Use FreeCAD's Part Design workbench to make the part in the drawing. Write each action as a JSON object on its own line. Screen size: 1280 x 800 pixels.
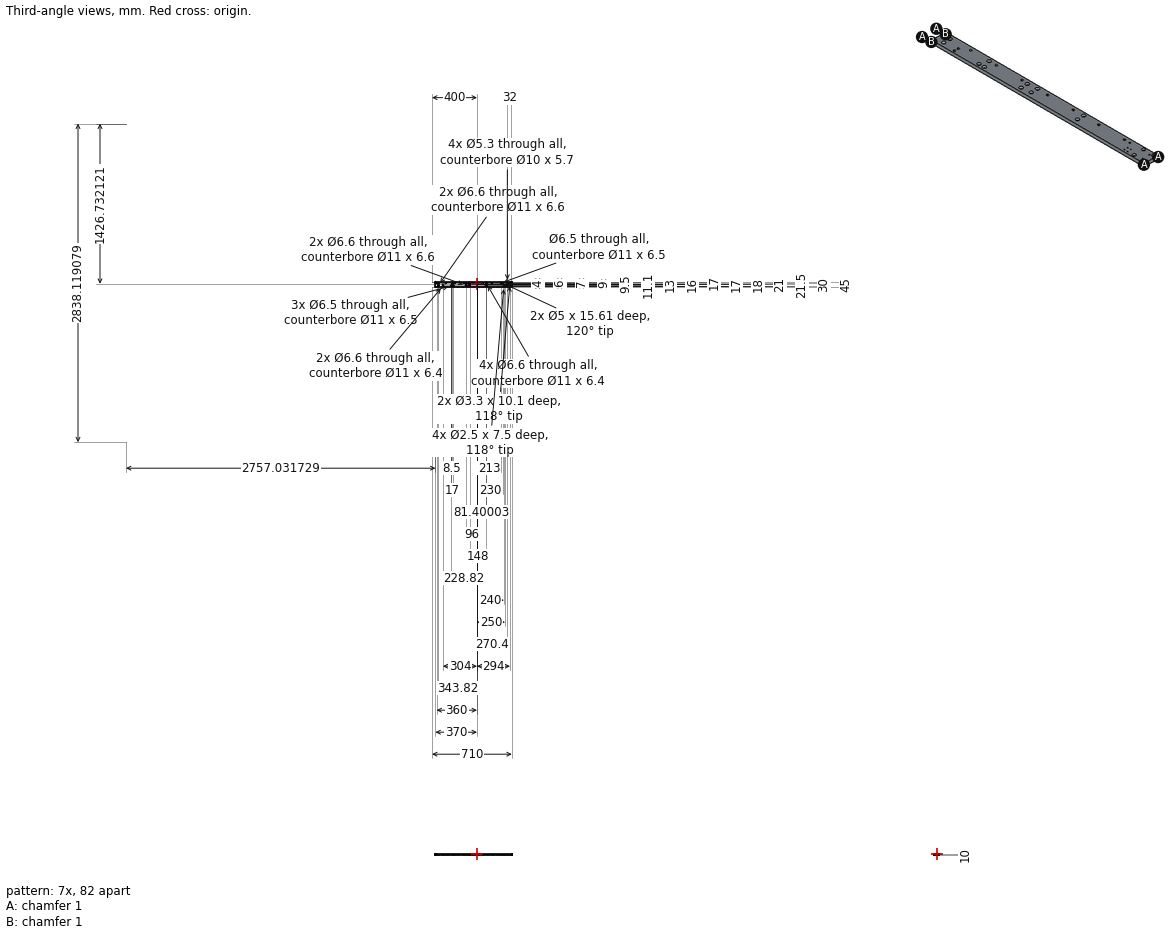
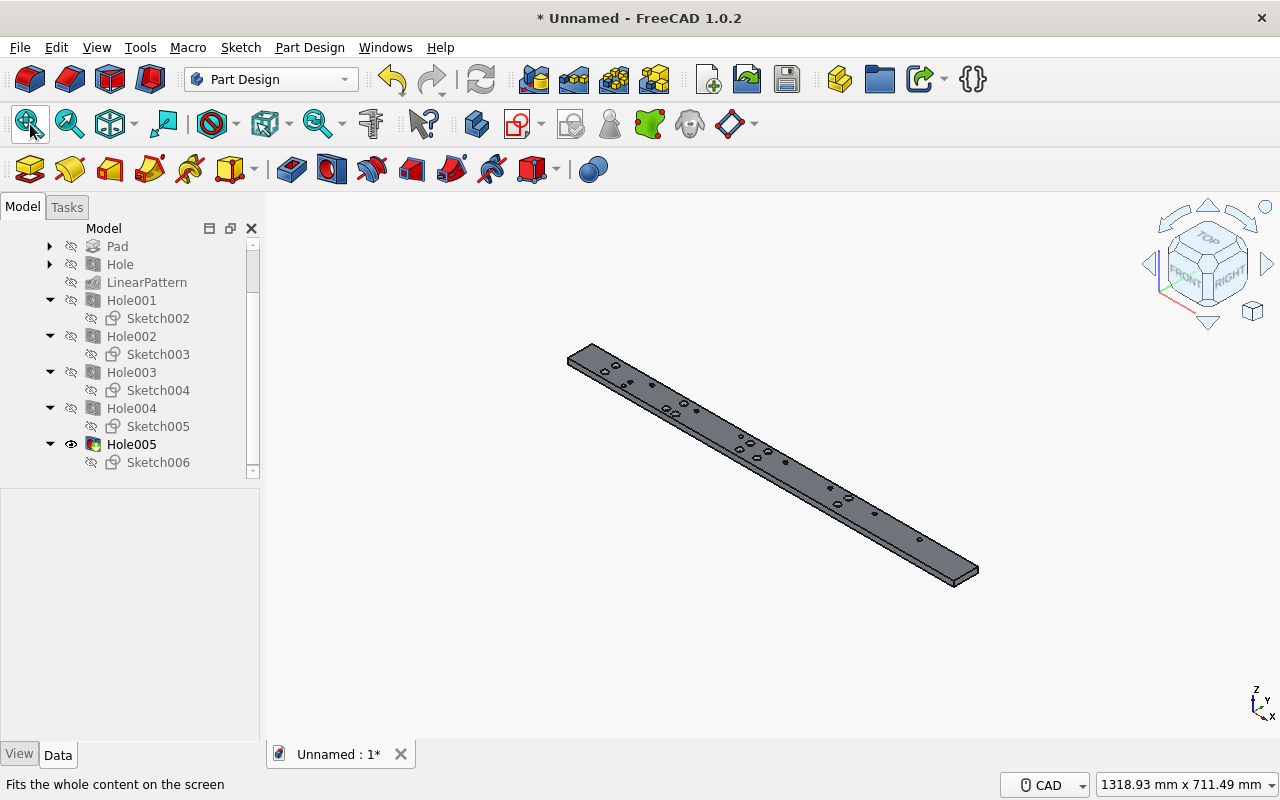
{"action": "left_click", "coordinate": [30, 124]}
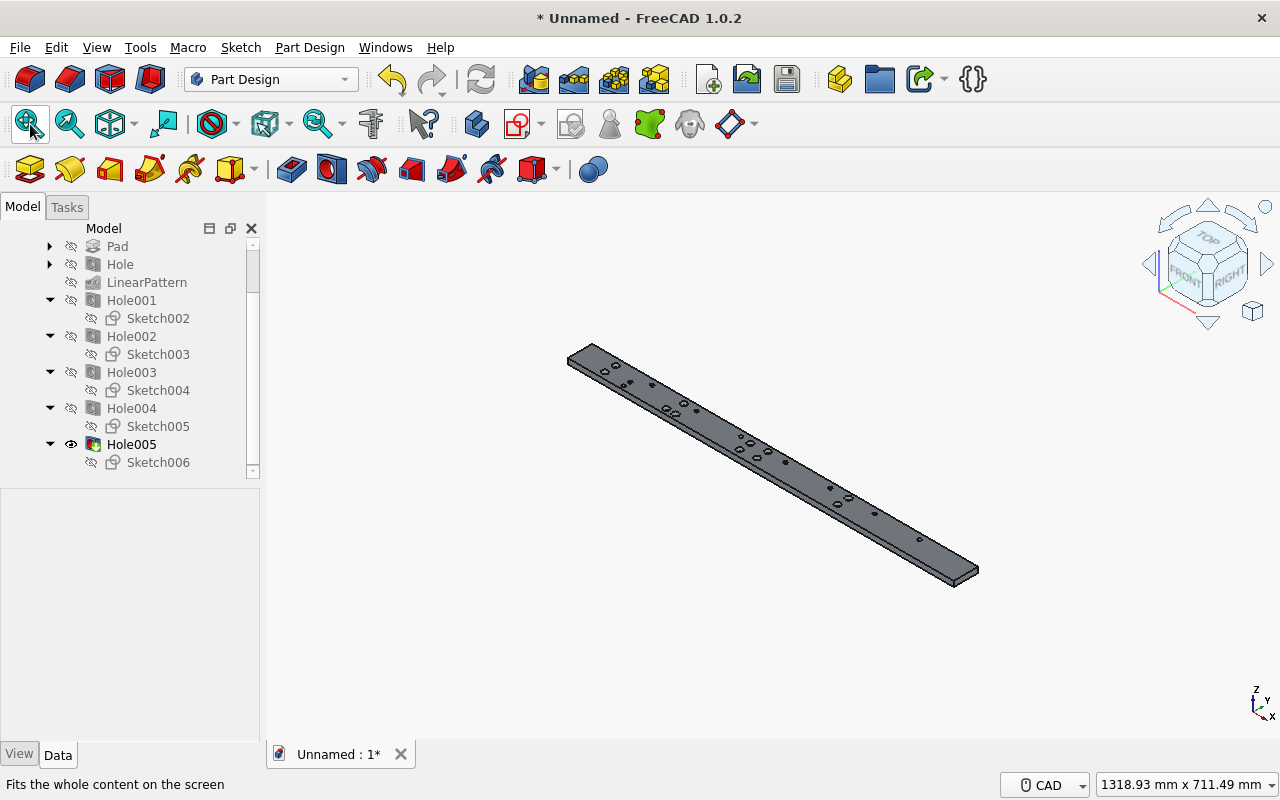
{"action": "scroll", "coordinate": [592, 346], "scroll_direction": "up", "scroll_amount": 9}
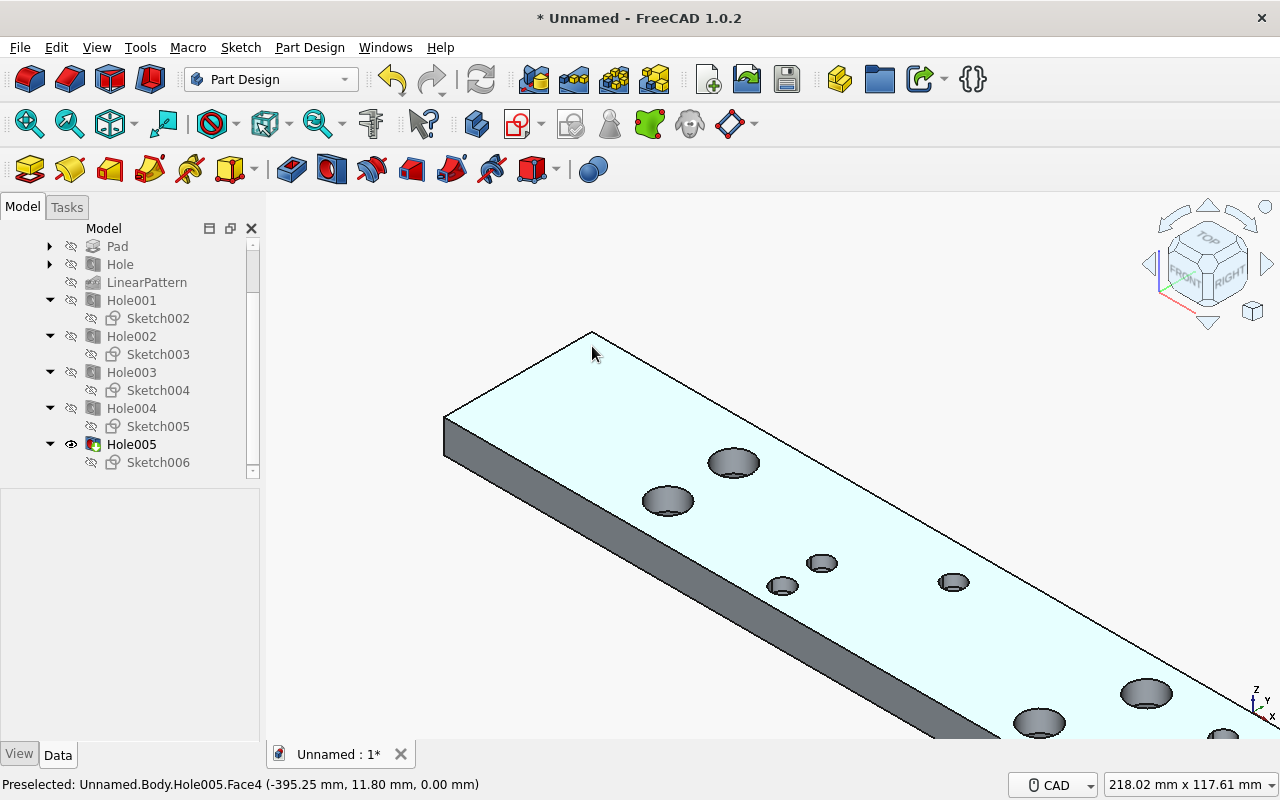
{"action": "left_click", "coordinate": [30, 124]}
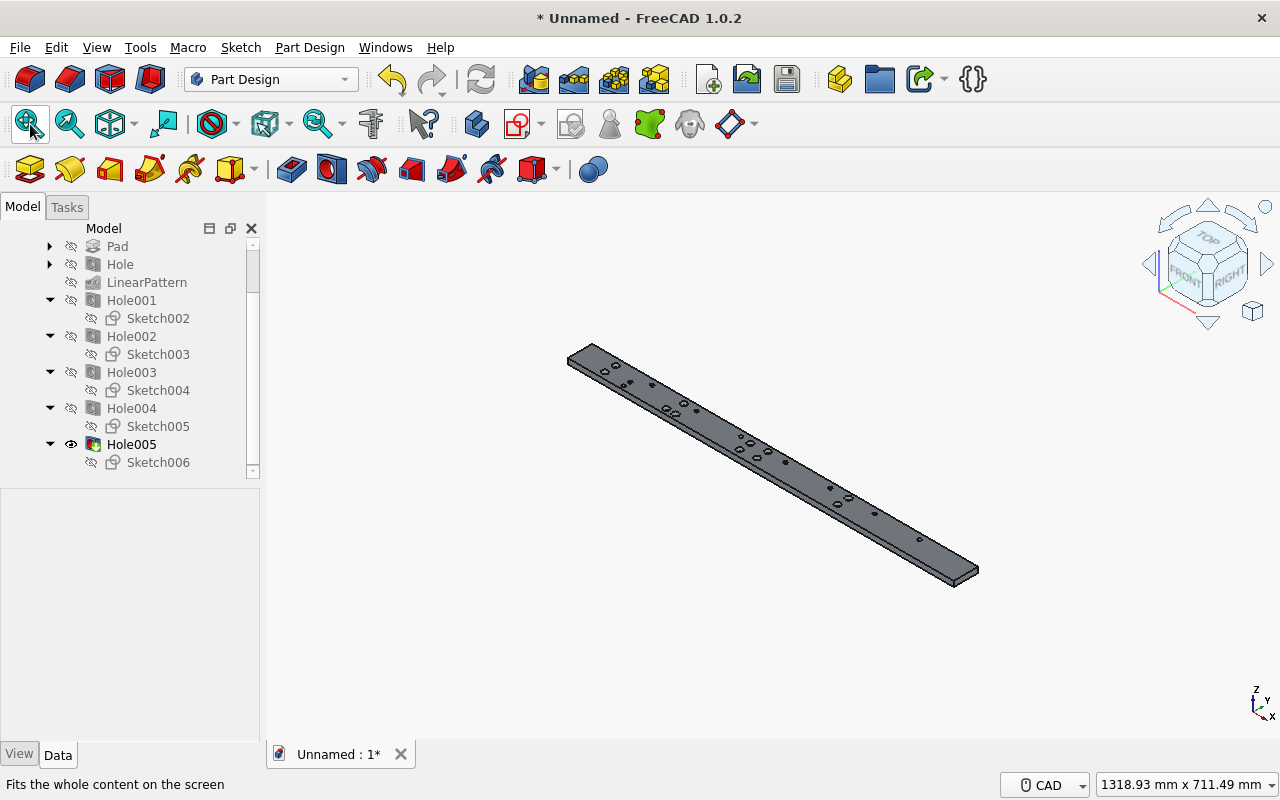
{"action": "key", "text": "1"}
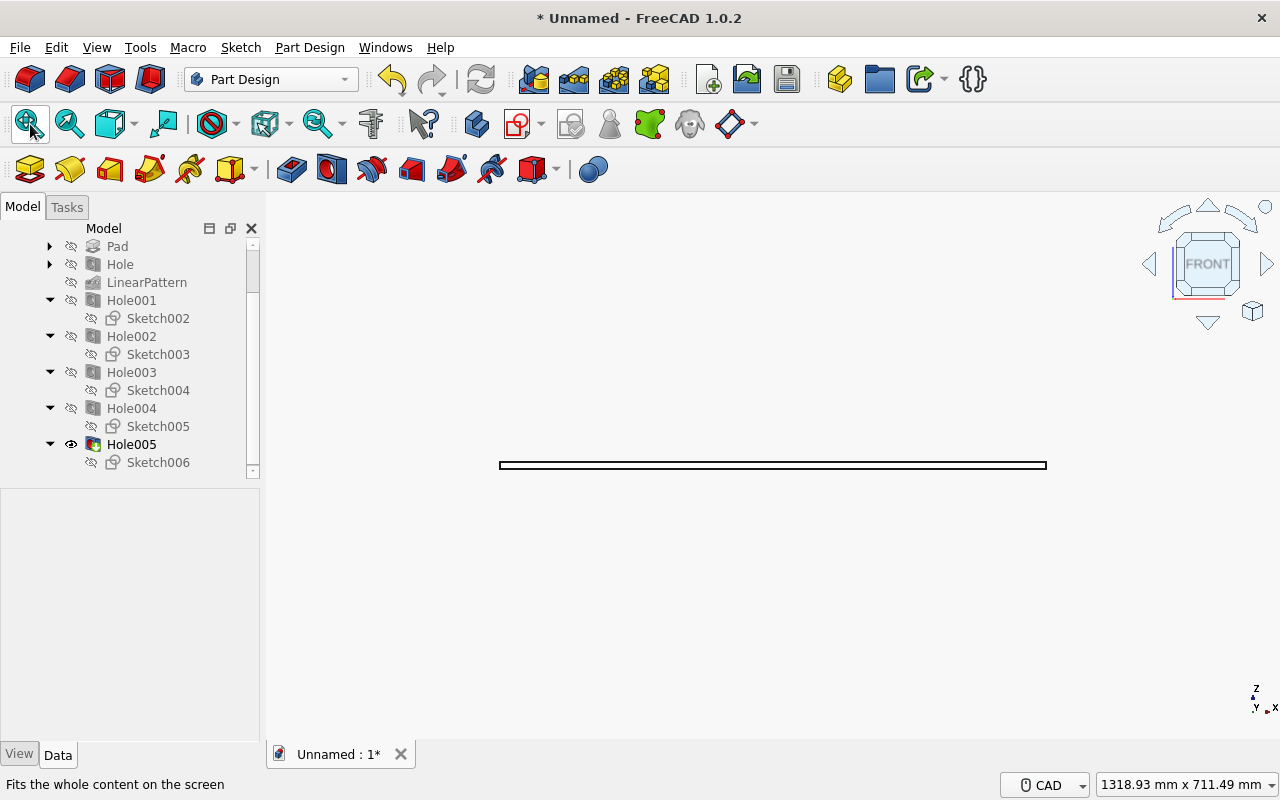
{"action": "scroll", "coordinate": [500, 465], "scroll_direction": "up", "scroll_amount": 9}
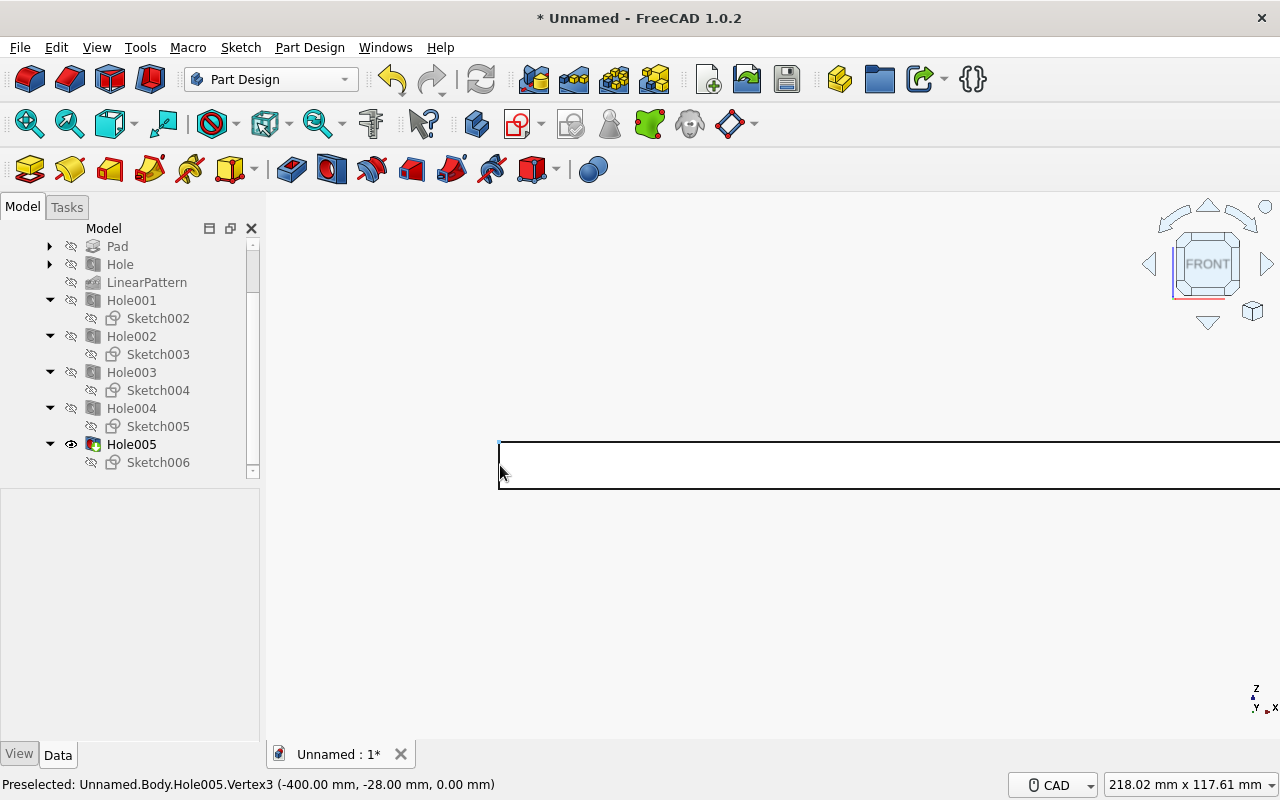
{"action": "left_click", "coordinate": [499, 465]}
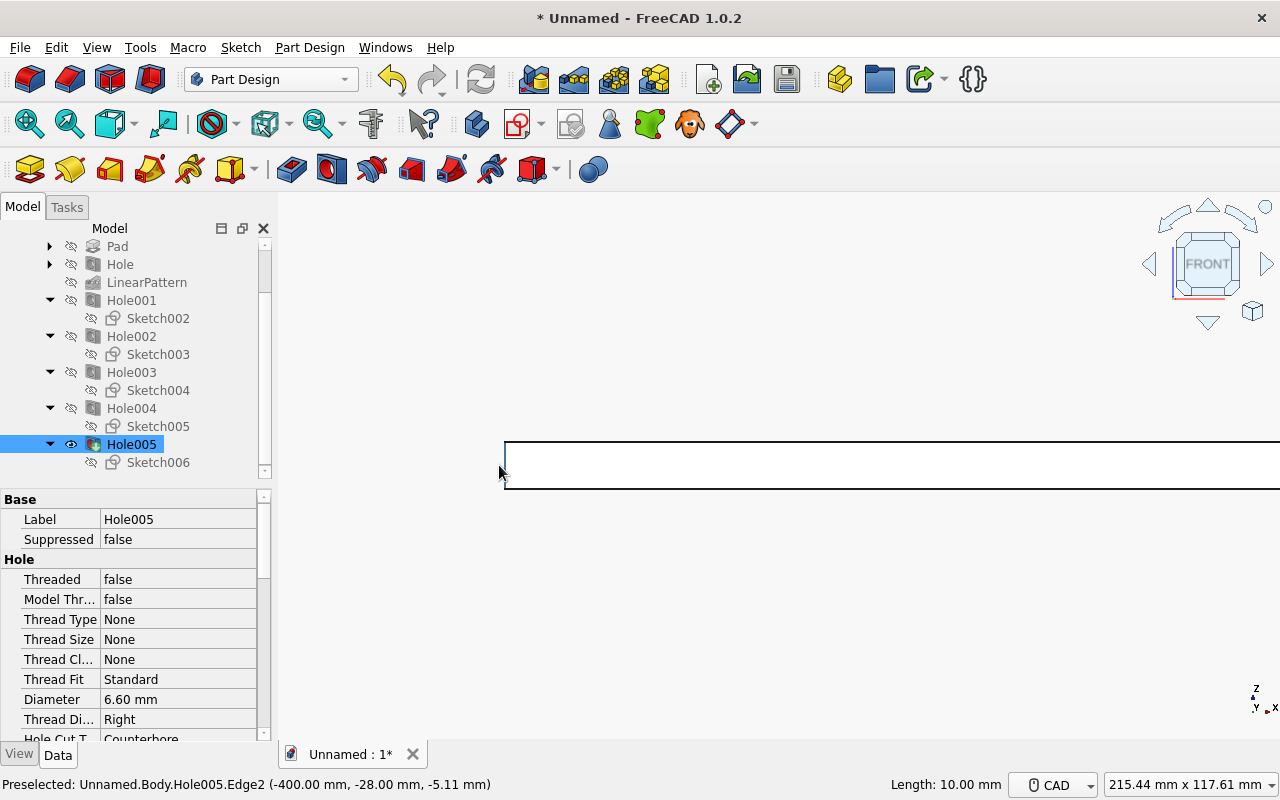
{"action": "left_click", "coordinate": [30, 124]}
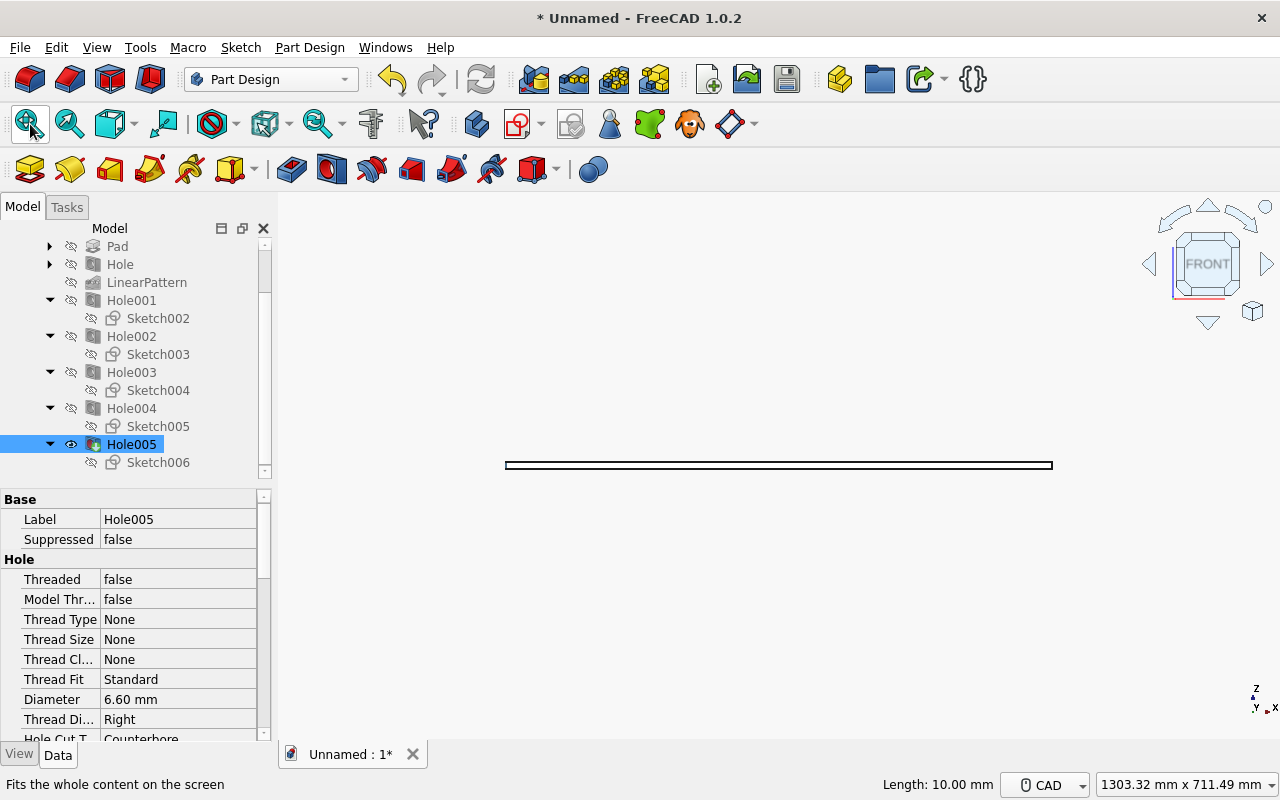
{"action": "key", "text": "3"}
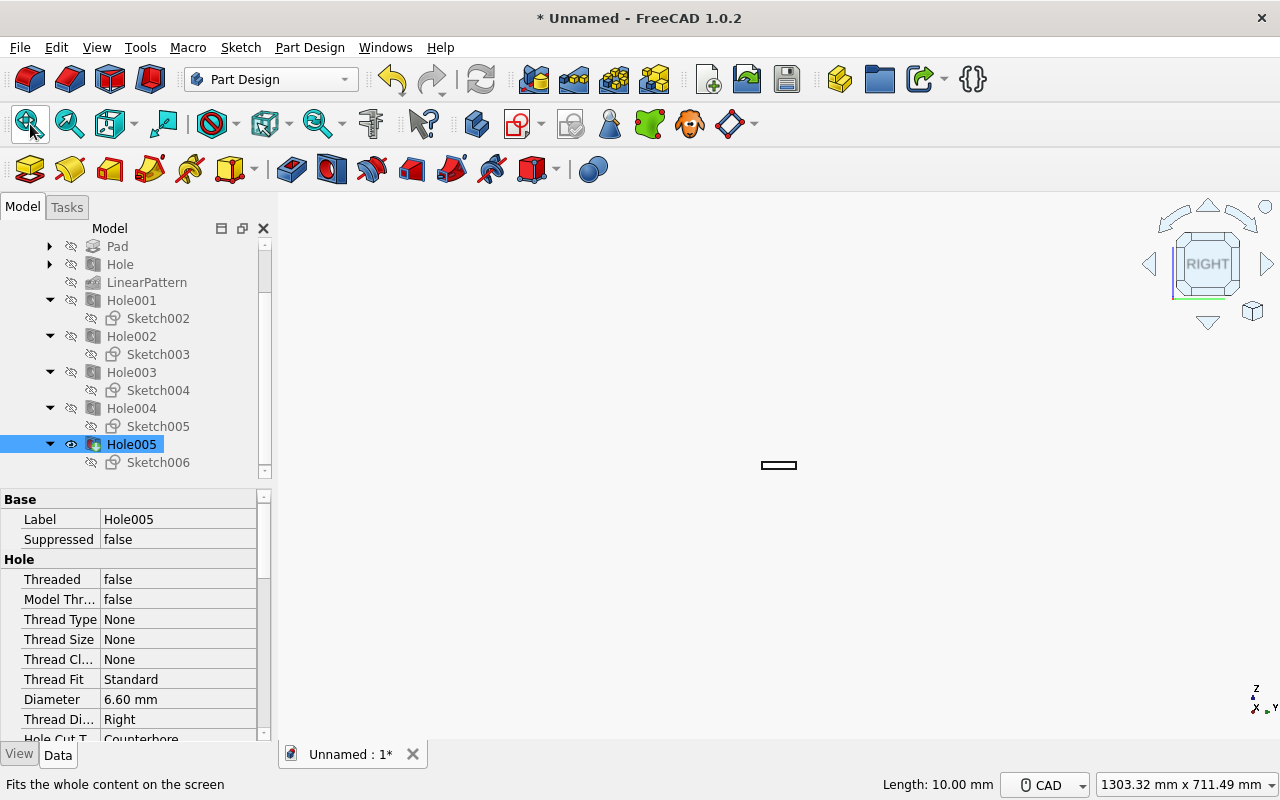
{"action": "left_click", "coordinate": [30, 124]}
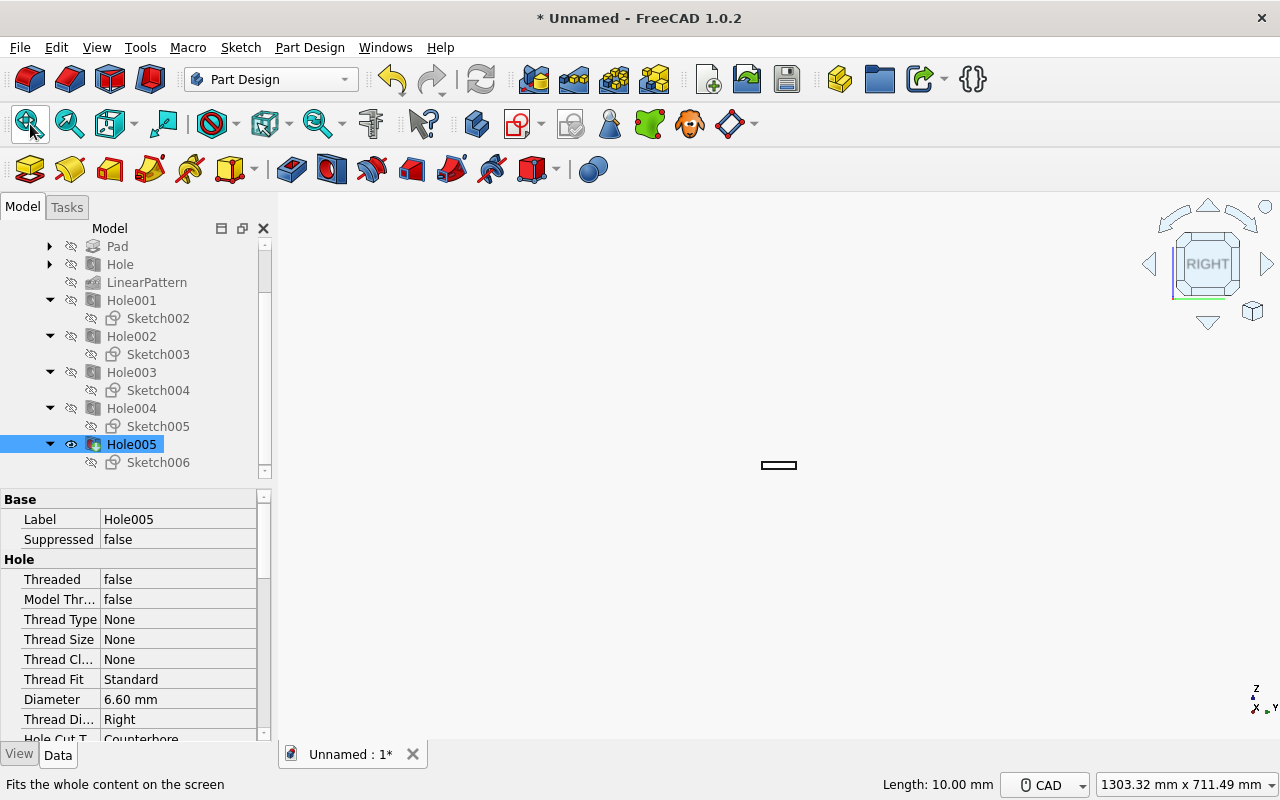
{"action": "scroll", "coordinate": [796, 464], "scroll_direction": "up", "scroll_amount": 9}